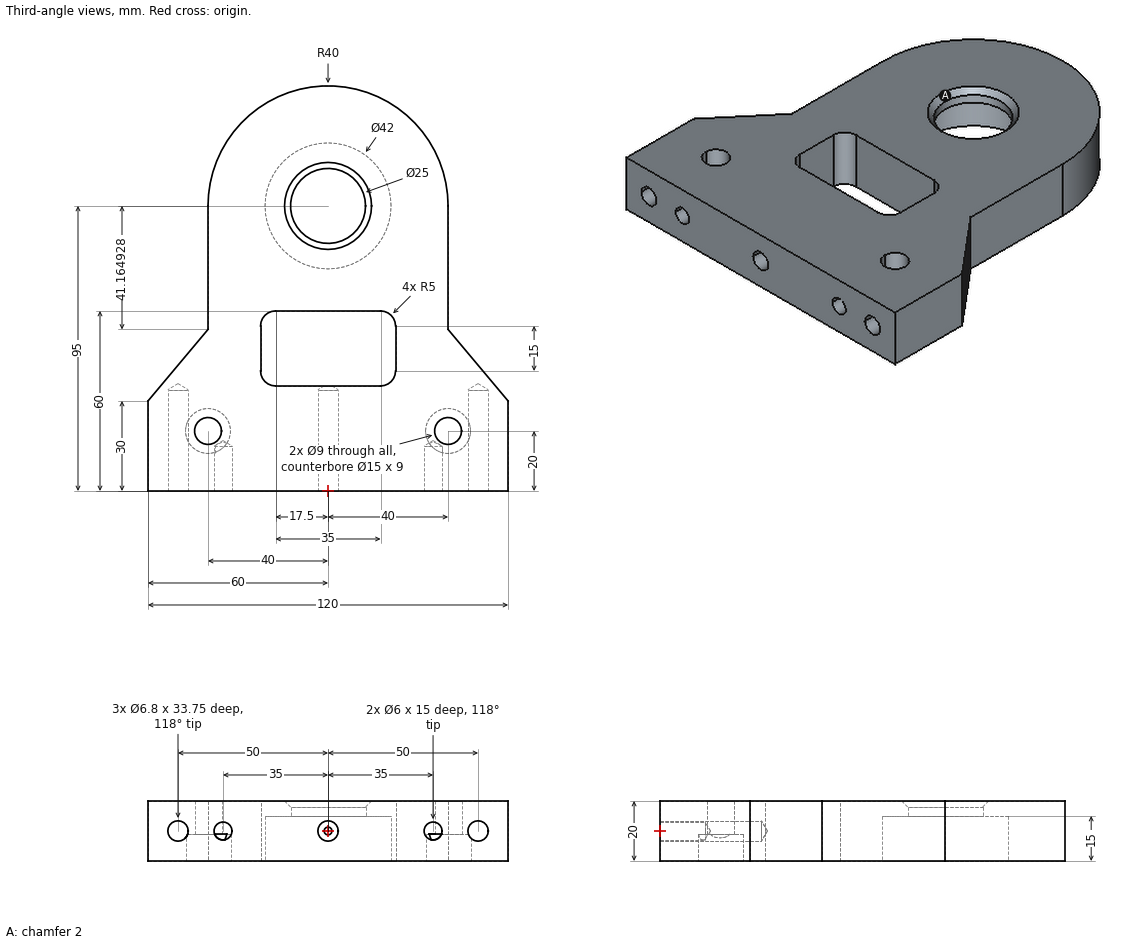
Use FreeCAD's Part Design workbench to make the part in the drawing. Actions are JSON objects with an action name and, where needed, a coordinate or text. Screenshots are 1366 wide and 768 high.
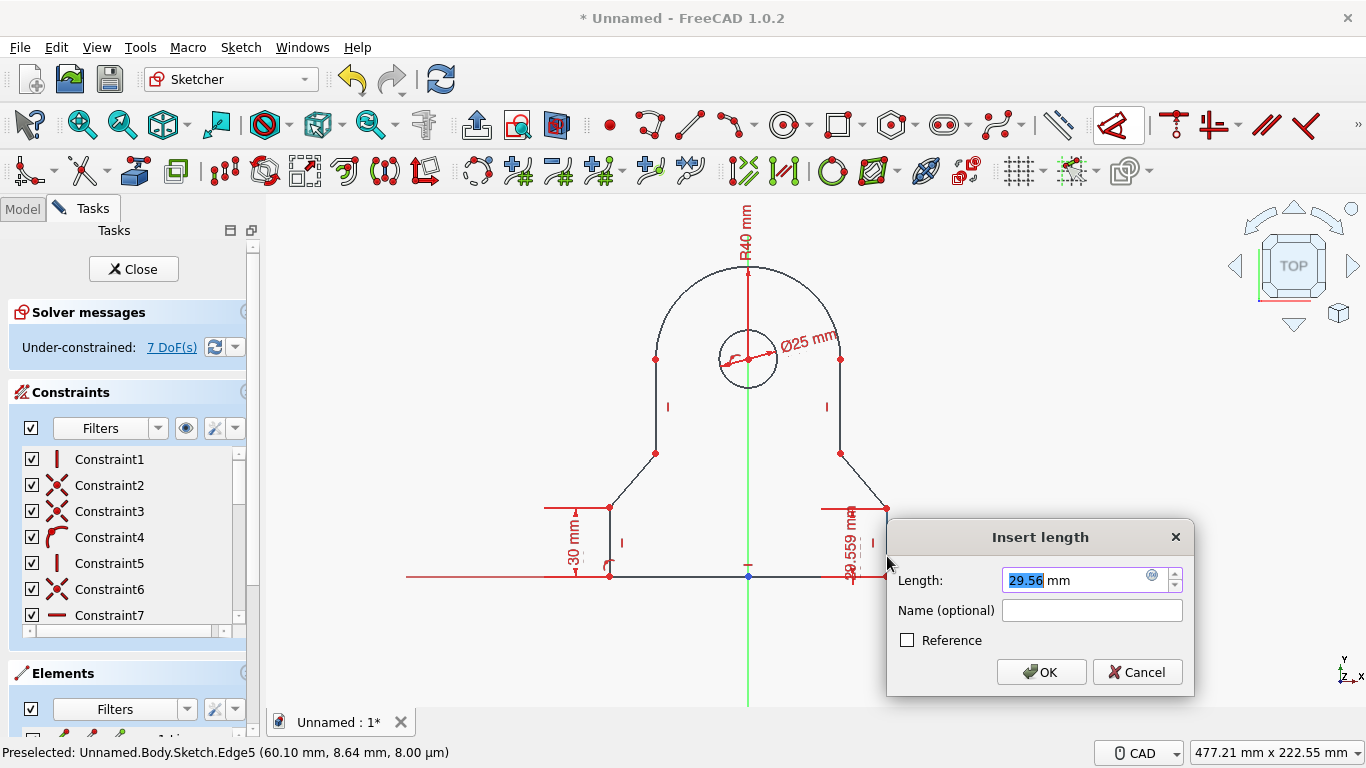
{"action": "type", "text": "30"}
{"action": "key", "text": "Return"}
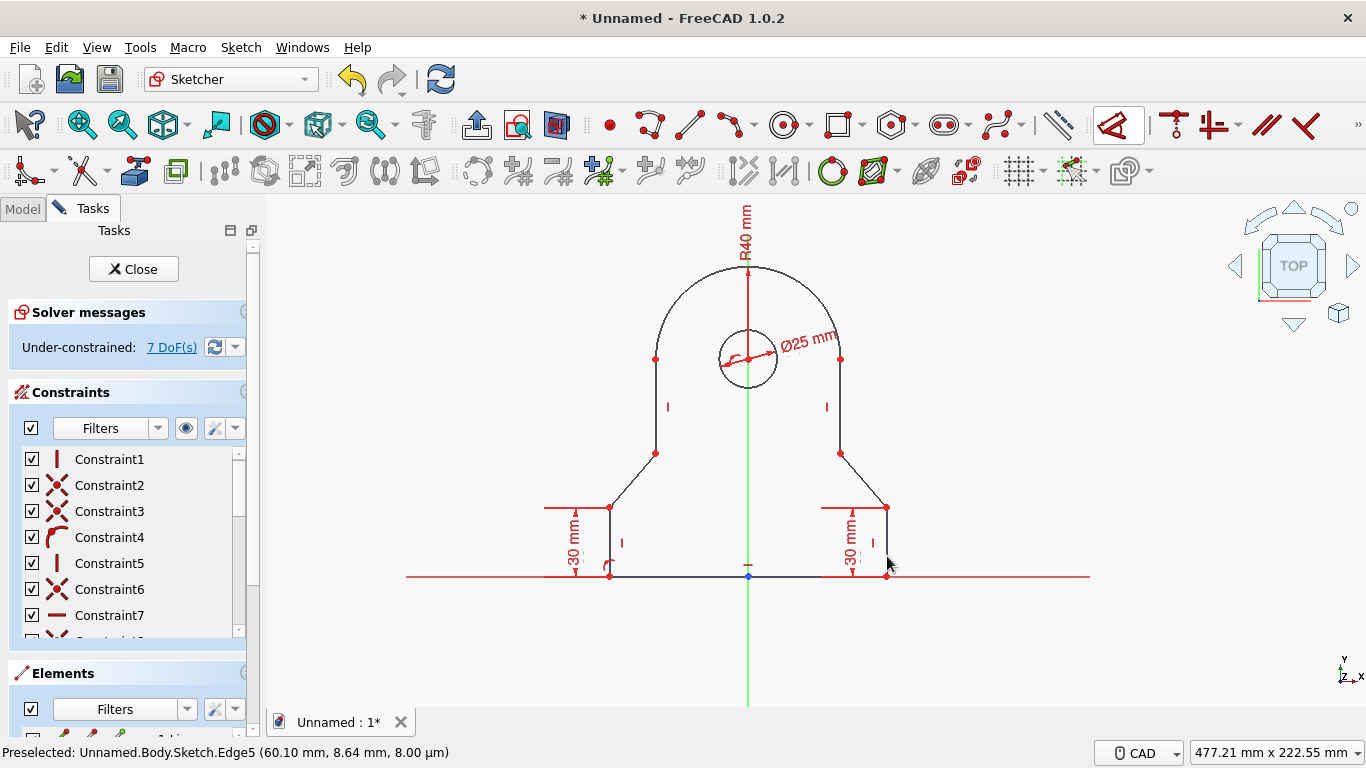
{"action": "left_click", "coordinate": [748, 359]}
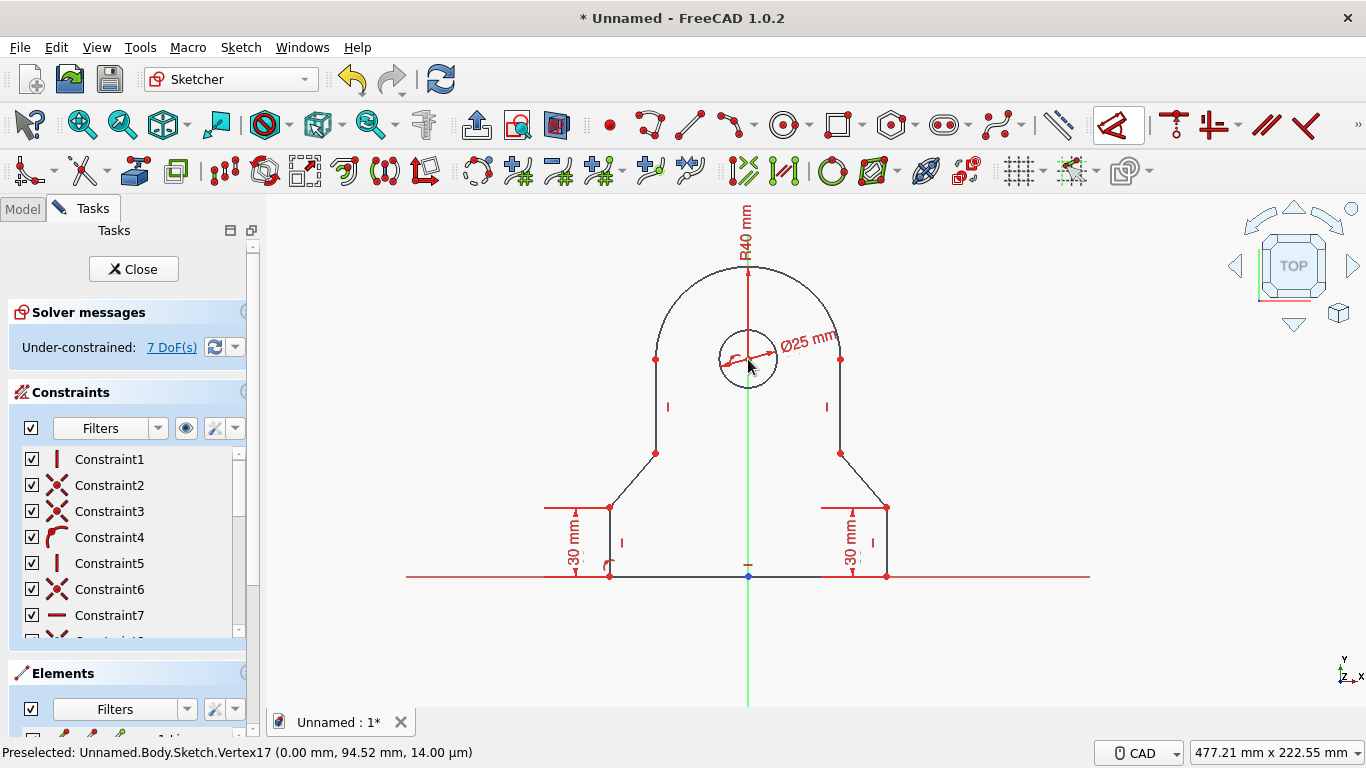
{"action": "left_click", "coordinate": [1138, 126]}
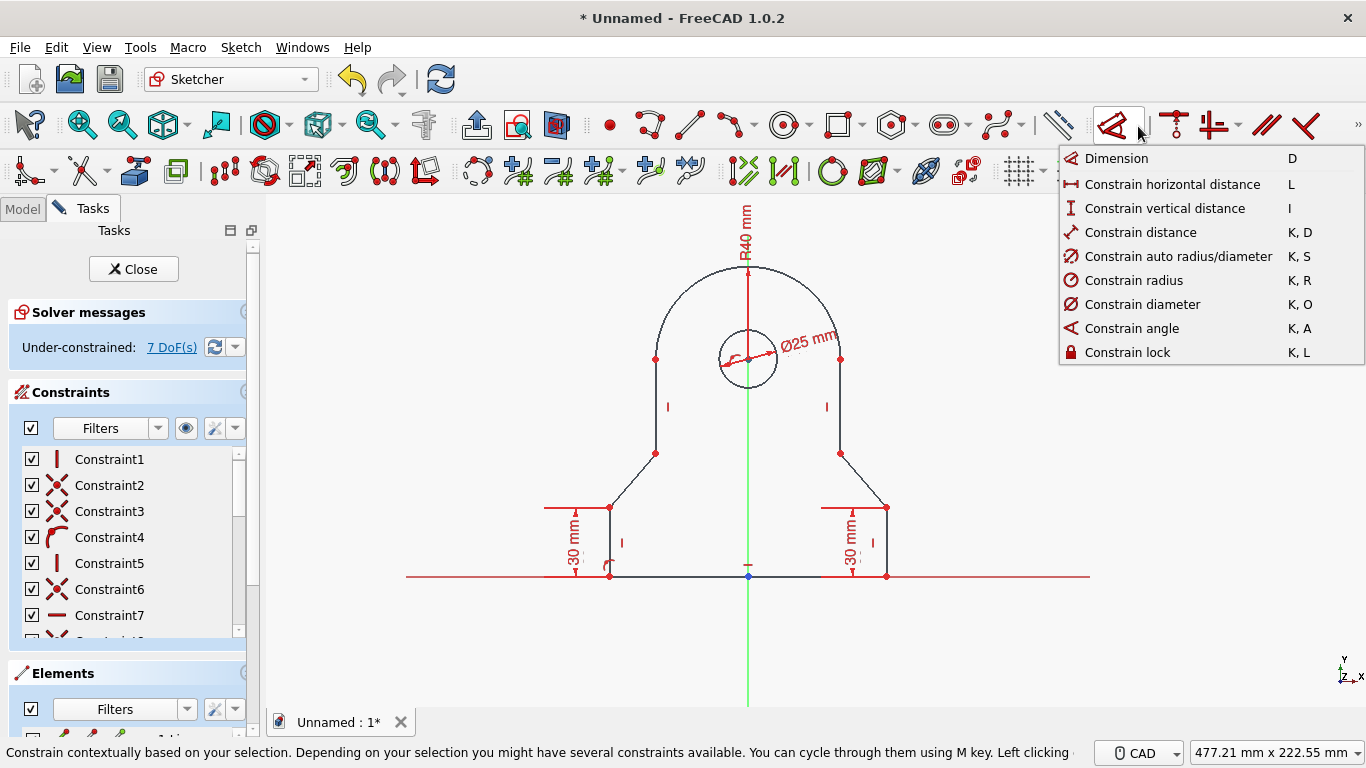
{"action": "left_click", "coordinate": [1212, 208]}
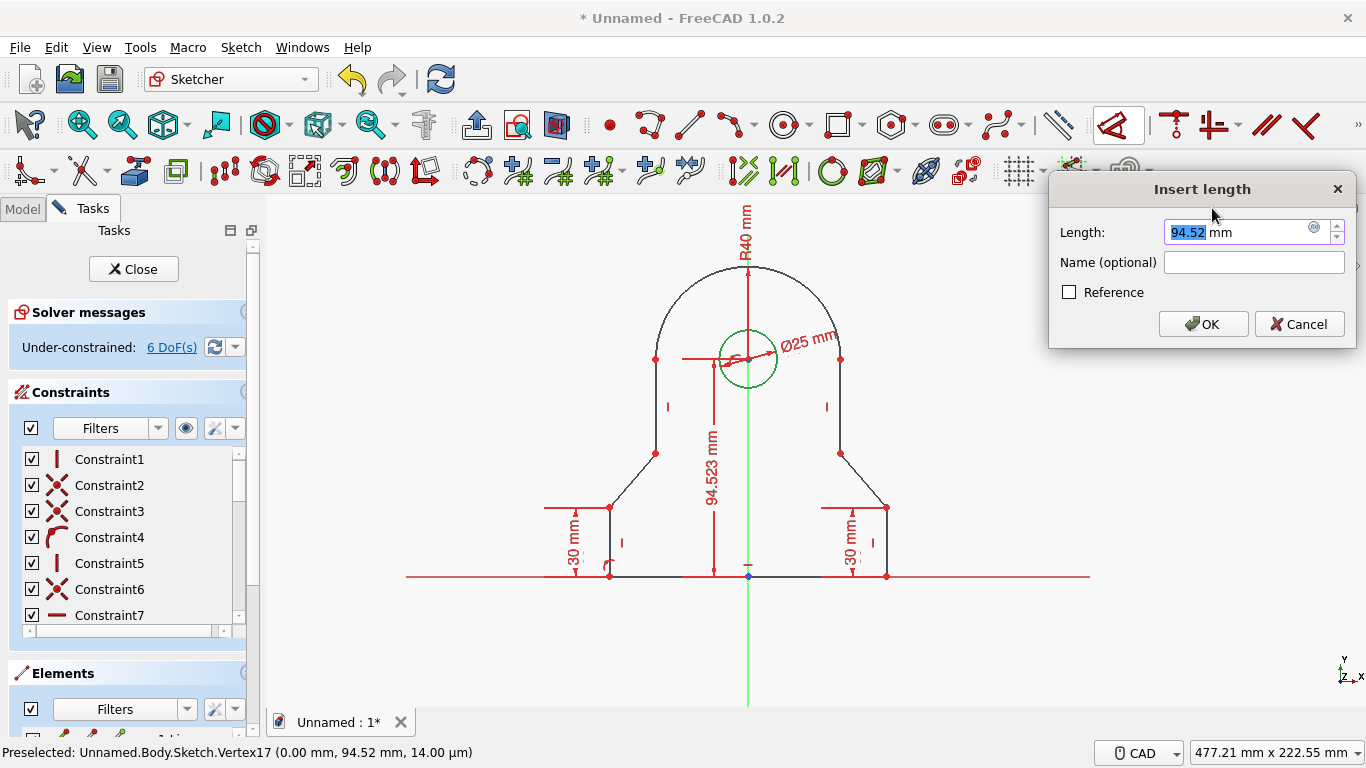
{"action": "type", "text": "95"}
{"action": "key", "text": "Return"}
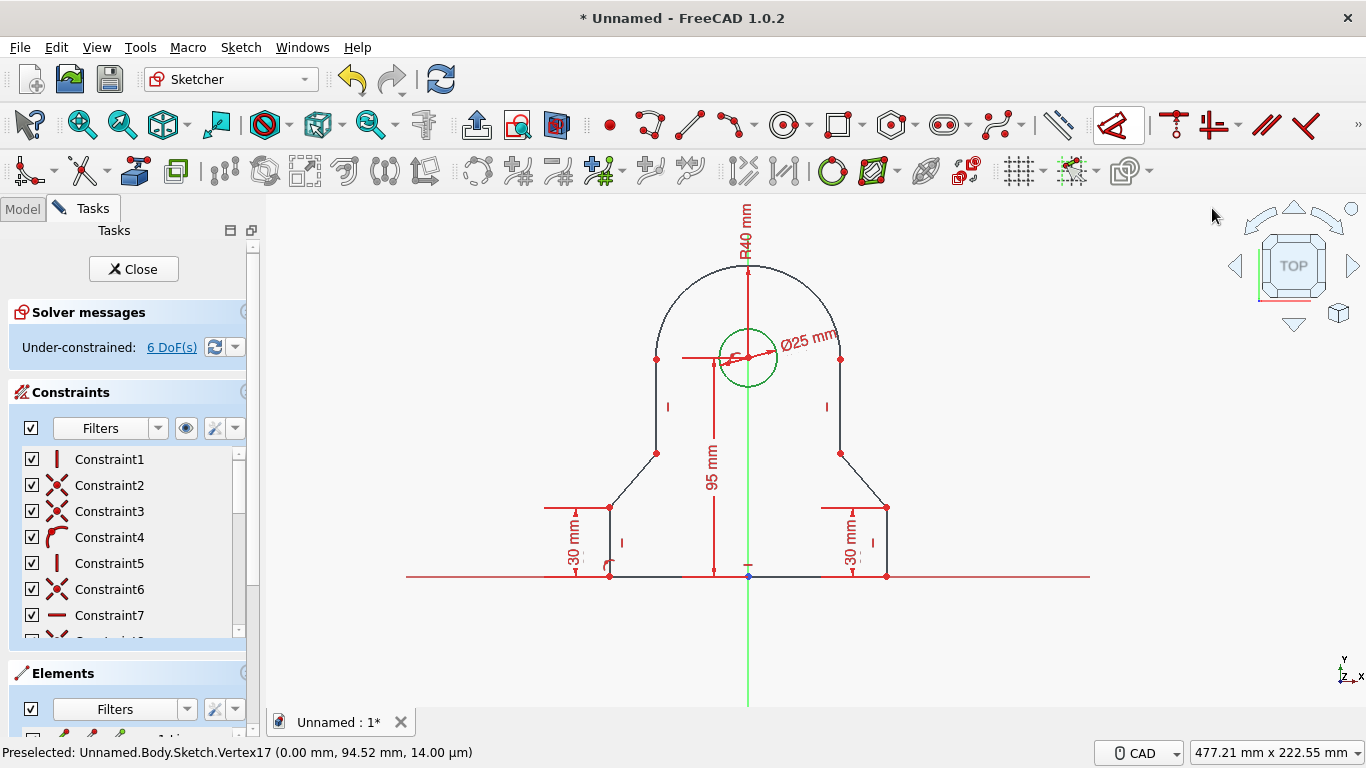
{"action": "left_click", "coordinate": [693, 577]}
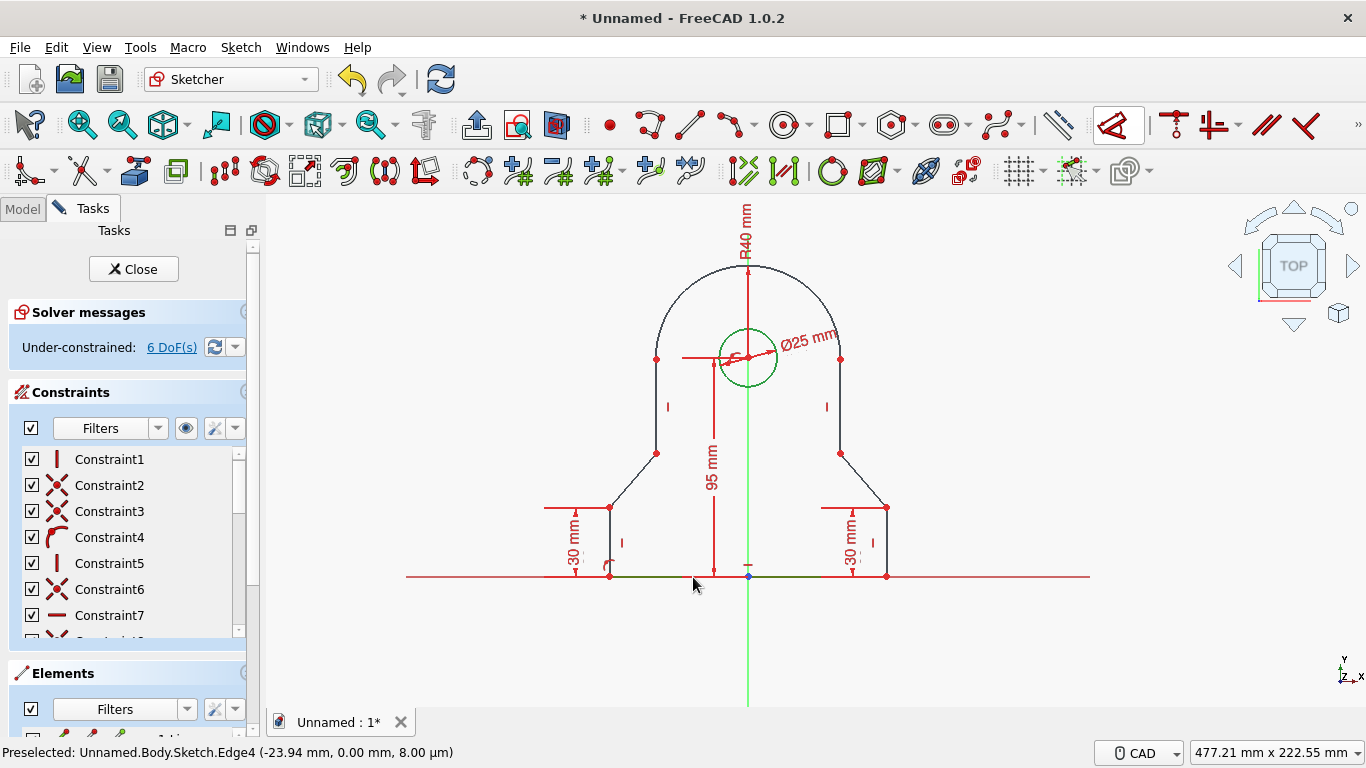
{"action": "left_click", "coordinate": [1138, 126]}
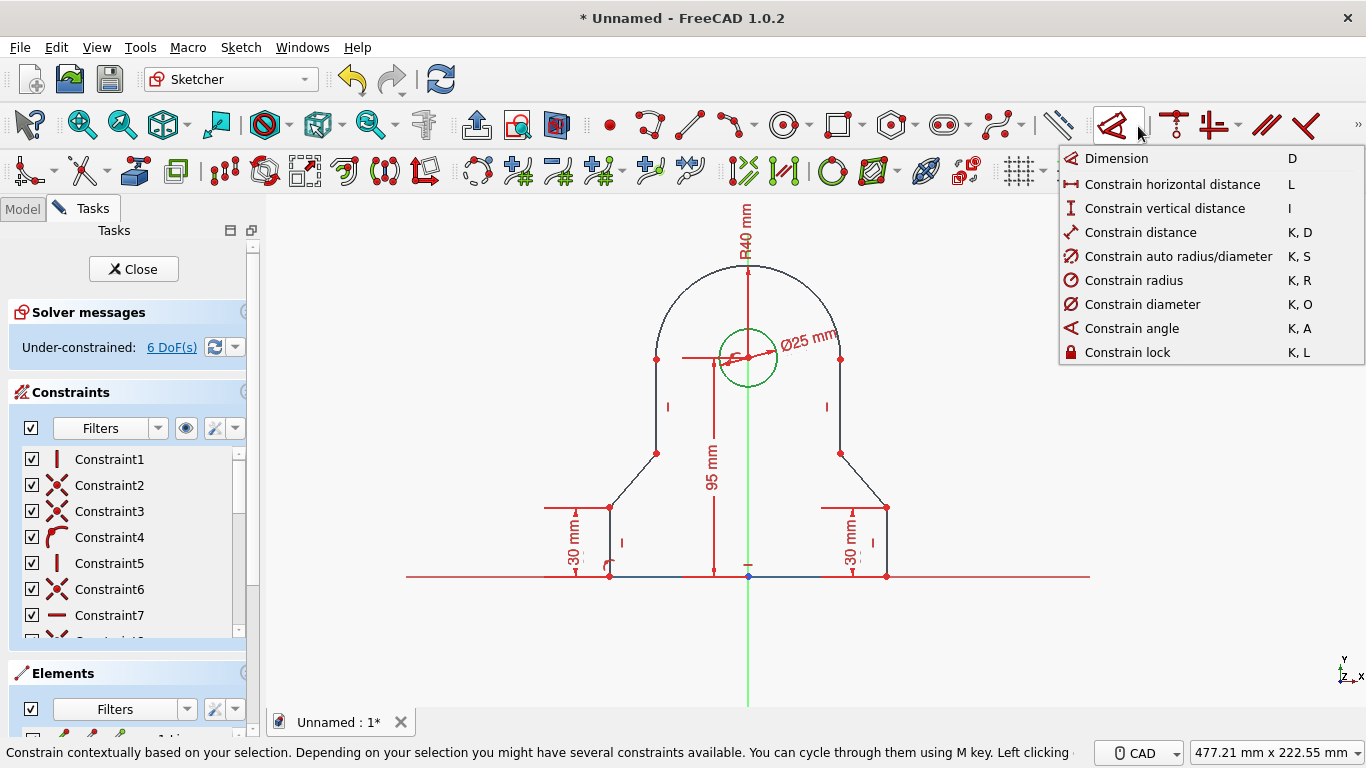
{"action": "left_click", "coordinate": [1212, 184]}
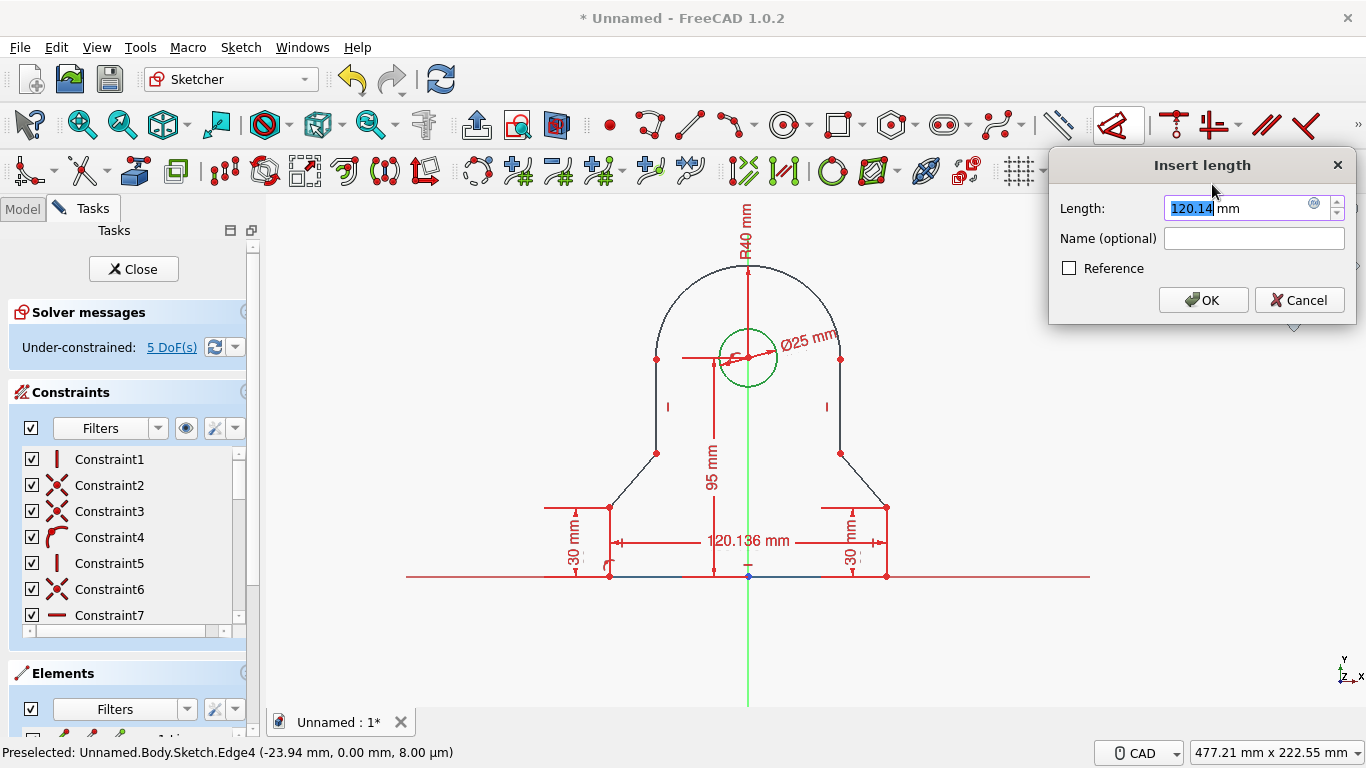
{"action": "type", "text": "120"}
{"action": "key", "text": "Return"}